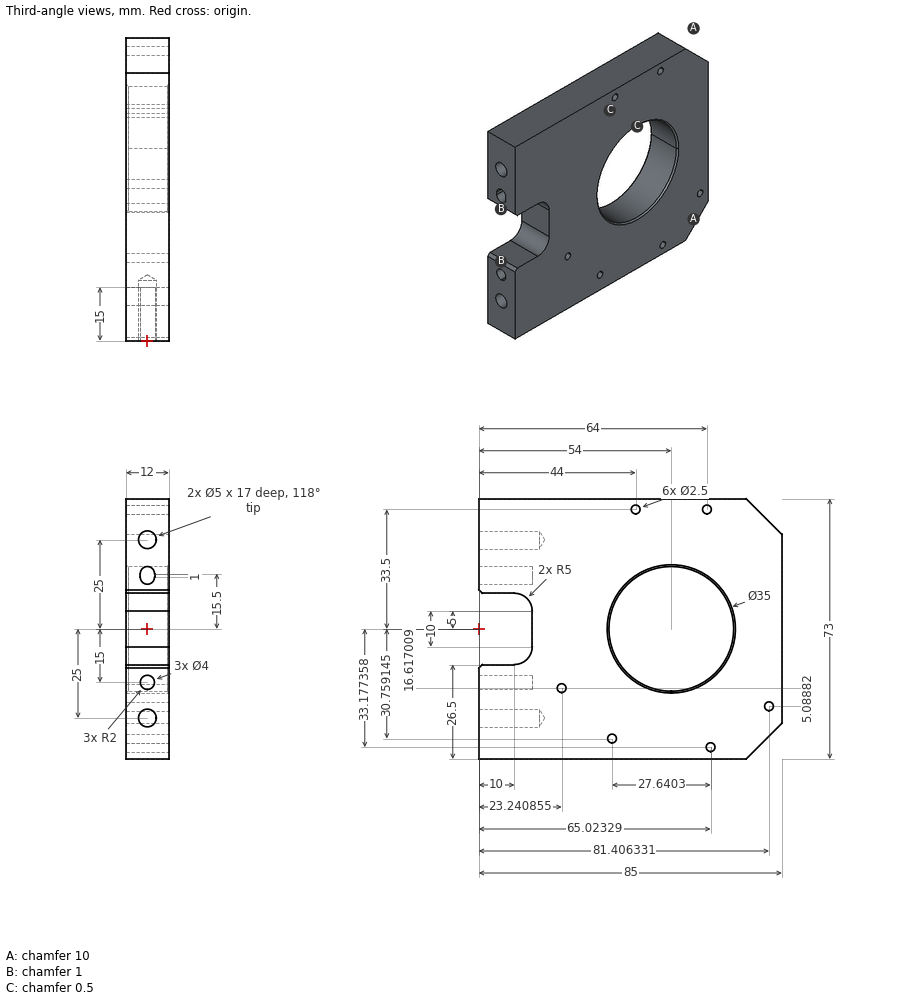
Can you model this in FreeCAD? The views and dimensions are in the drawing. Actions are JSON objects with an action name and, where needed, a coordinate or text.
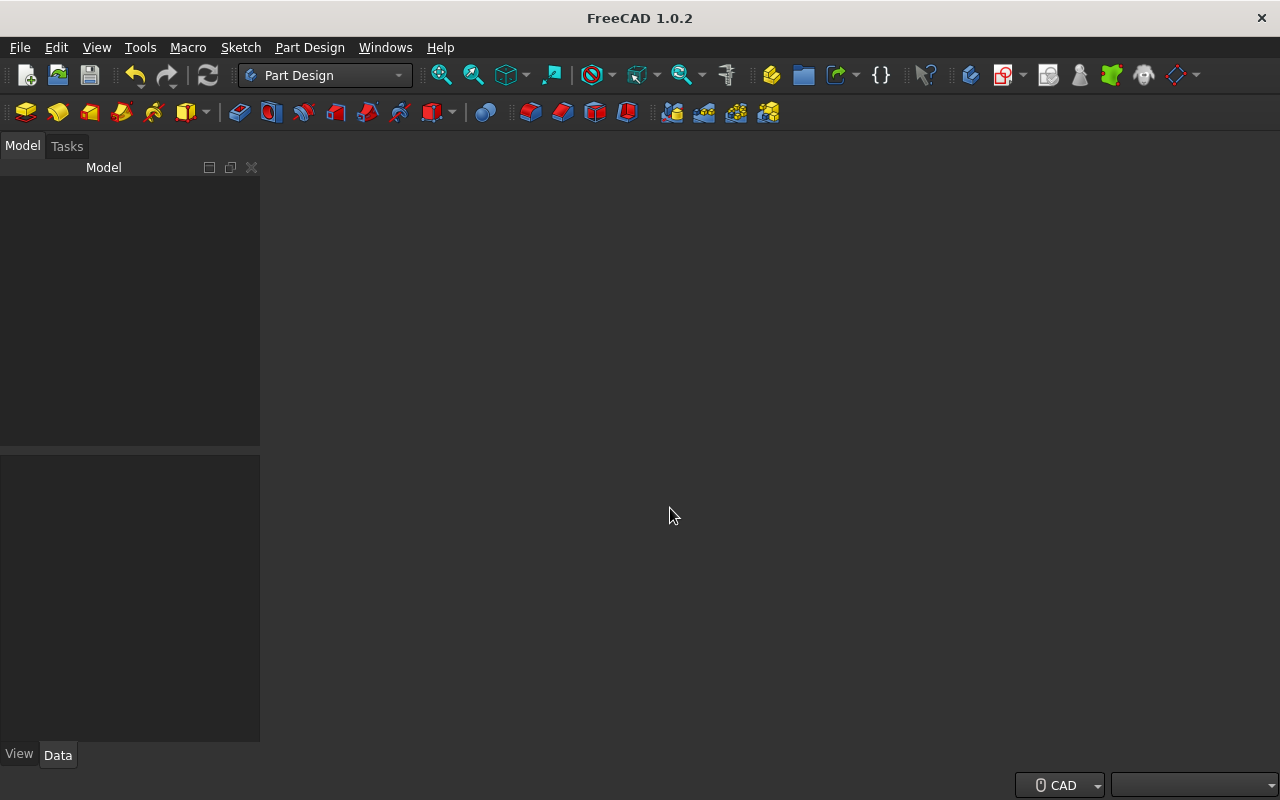
{"action": "left_click", "coordinate": [26, 76]}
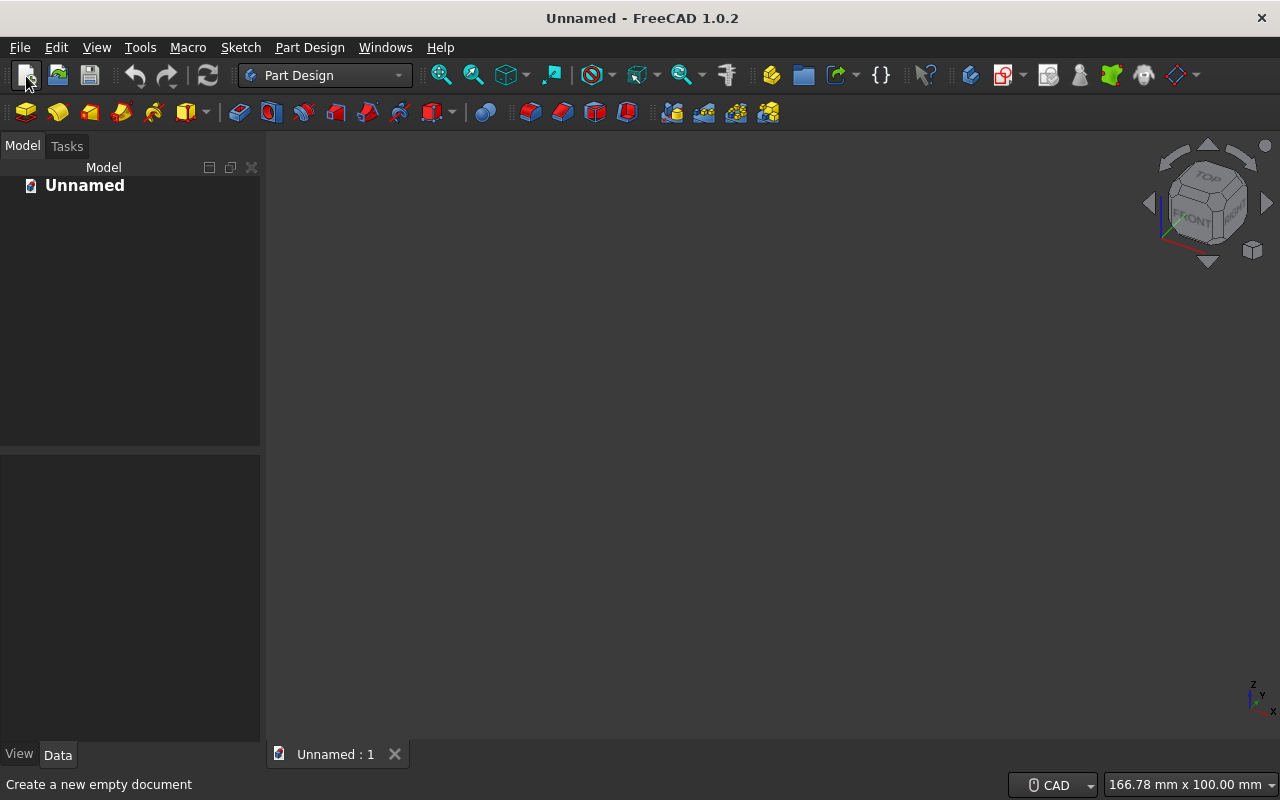
{"action": "left_click", "coordinate": [1004, 76]}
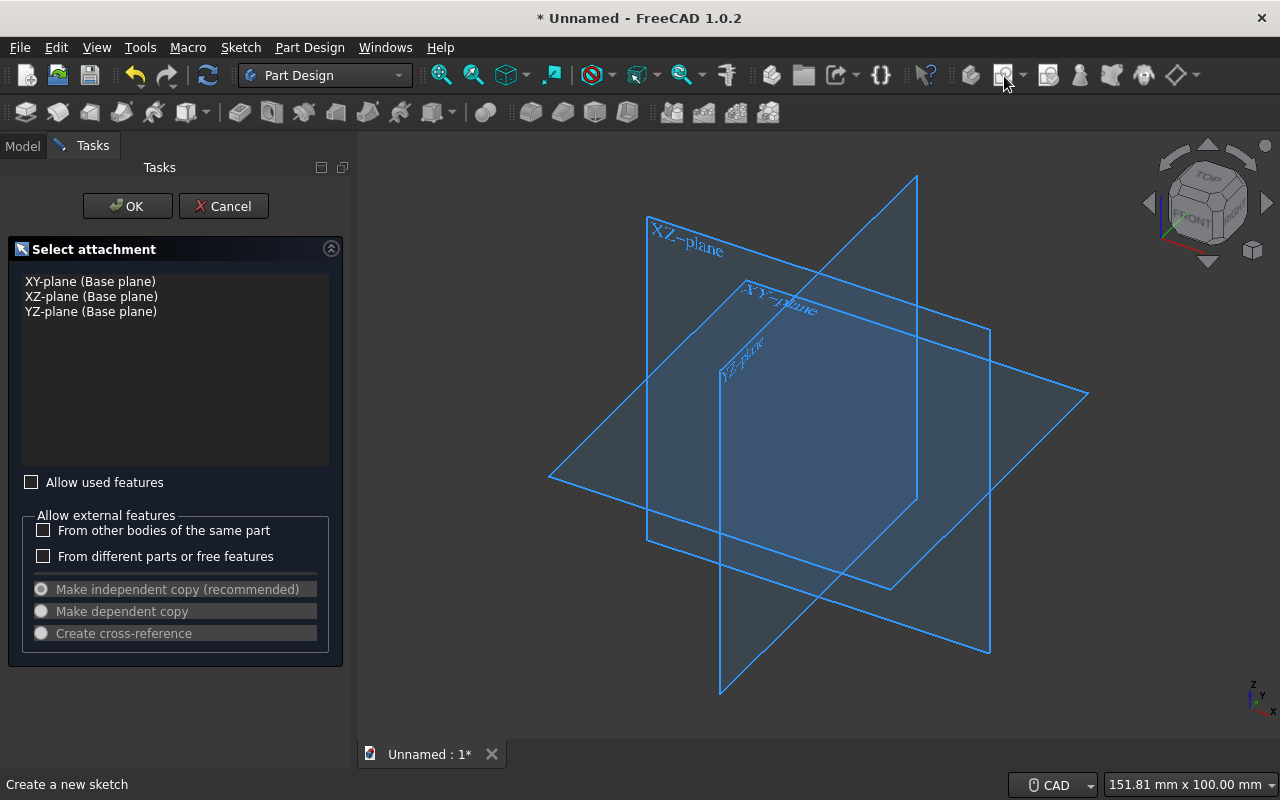
{"action": "left_click", "coordinate": [82, 312]}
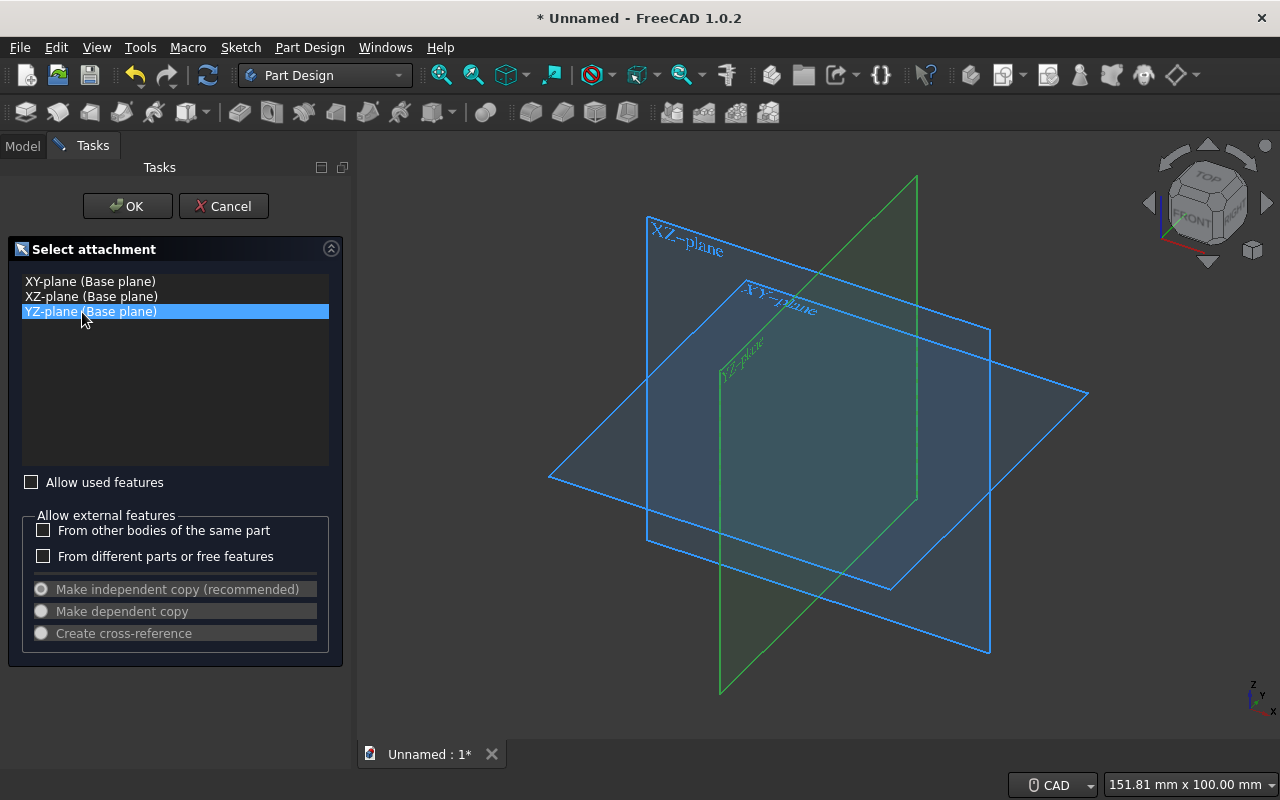
{"action": "left_click", "coordinate": [128, 206]}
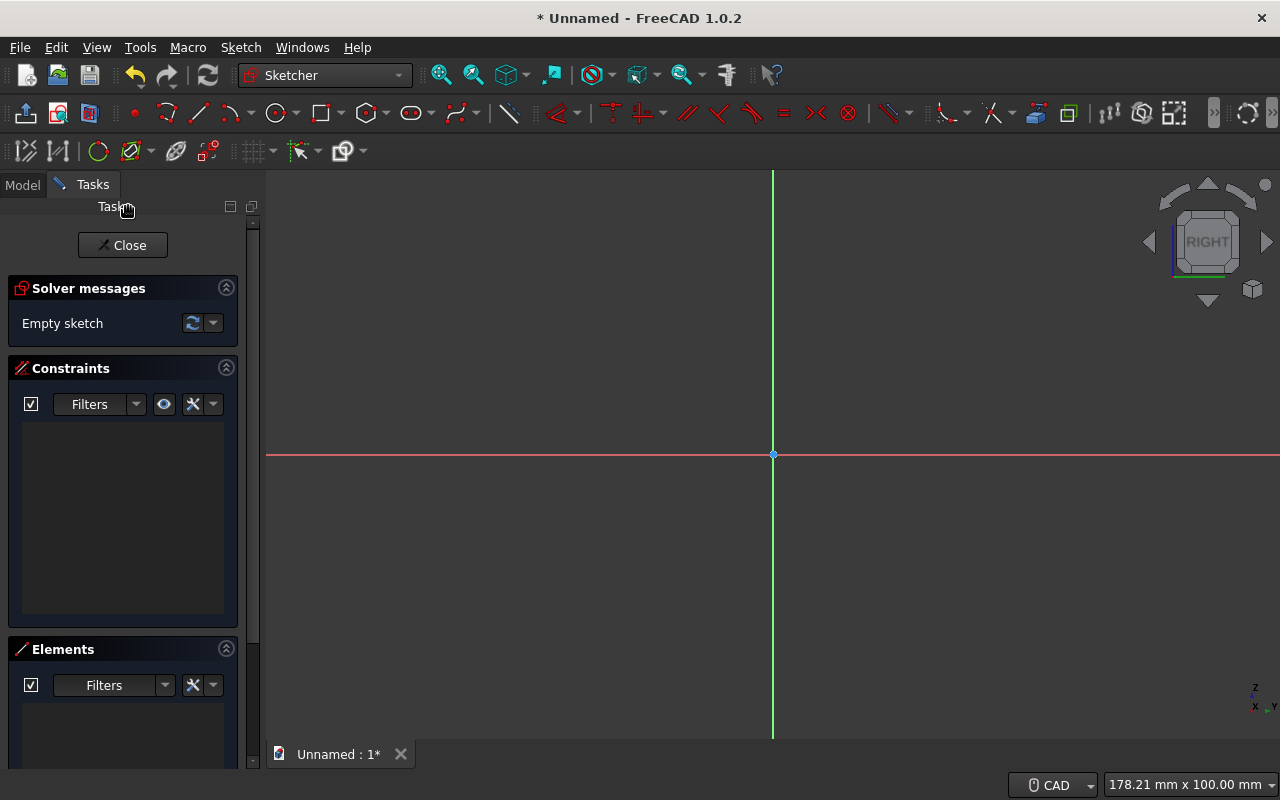
{"action": "scroll", "coordinate": [294, 455], "scroll_direction": "down", "scroll_amount": 1}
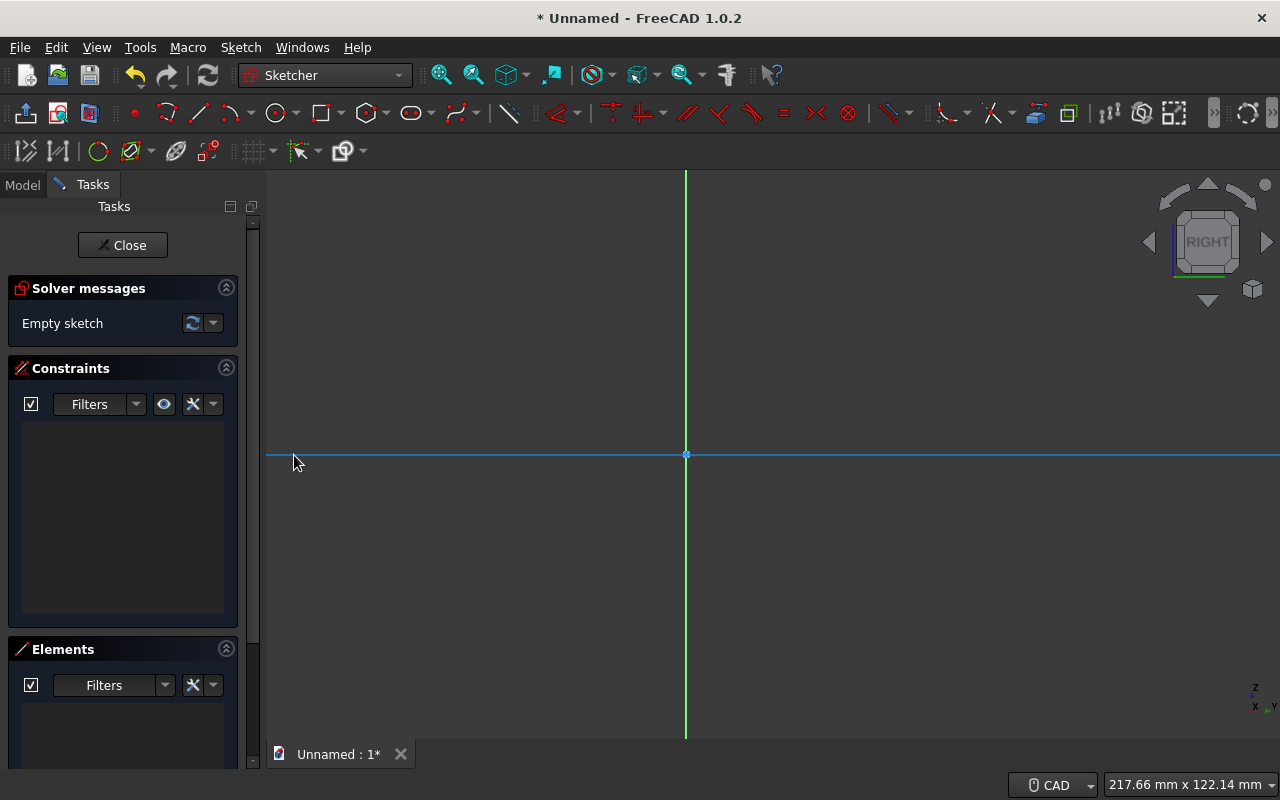
{"action": "left_click", "coordinate": [200, 114]}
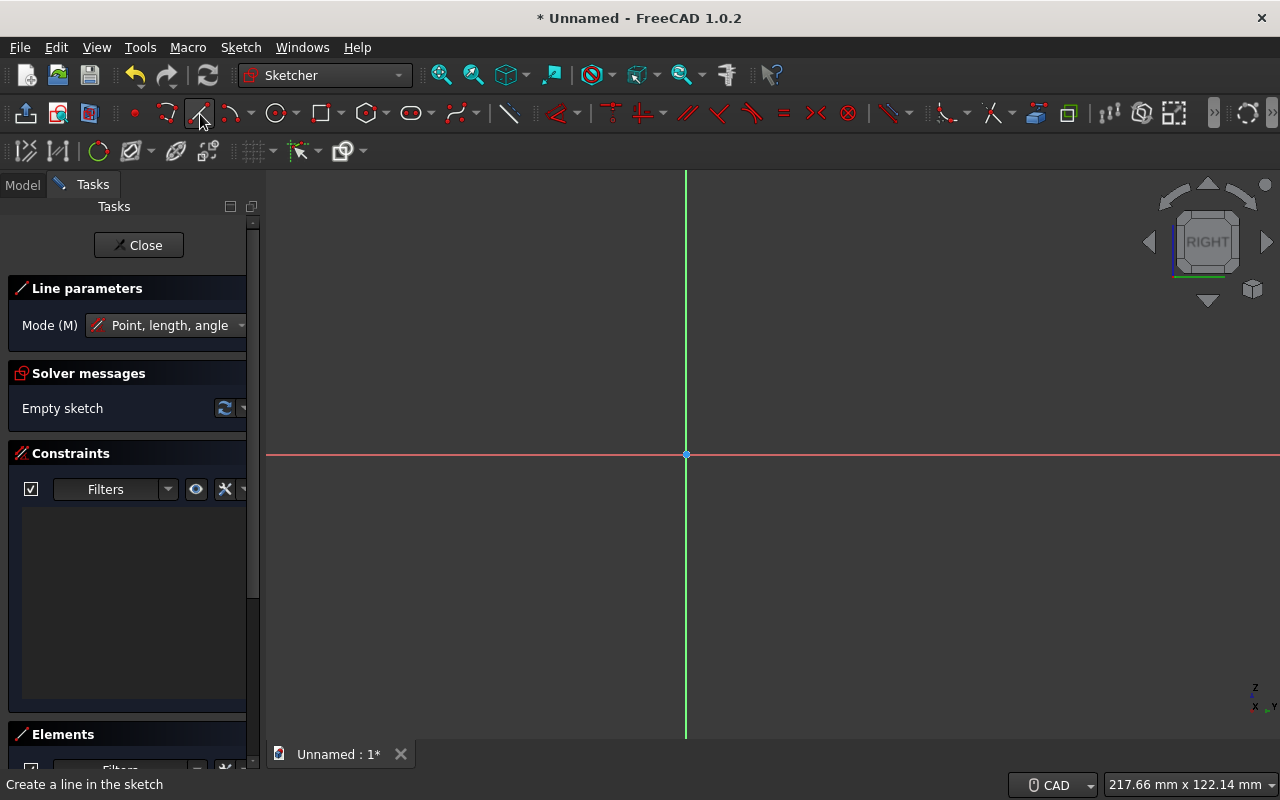
{"action": "left_click", "coordinate": [756, 431]}
{"action": "left_click", "coordinate": [756, 478]}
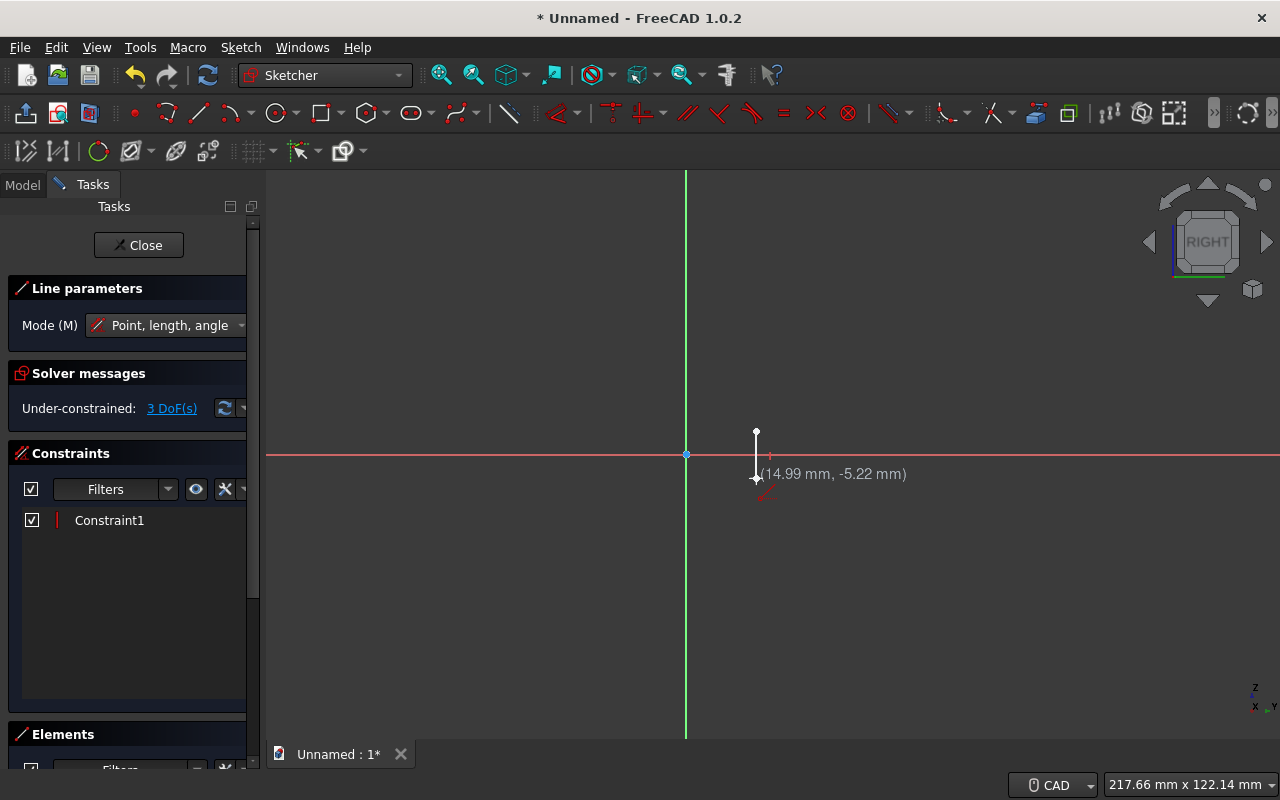
{"action": "left_click", "coordinate": [168, 114]}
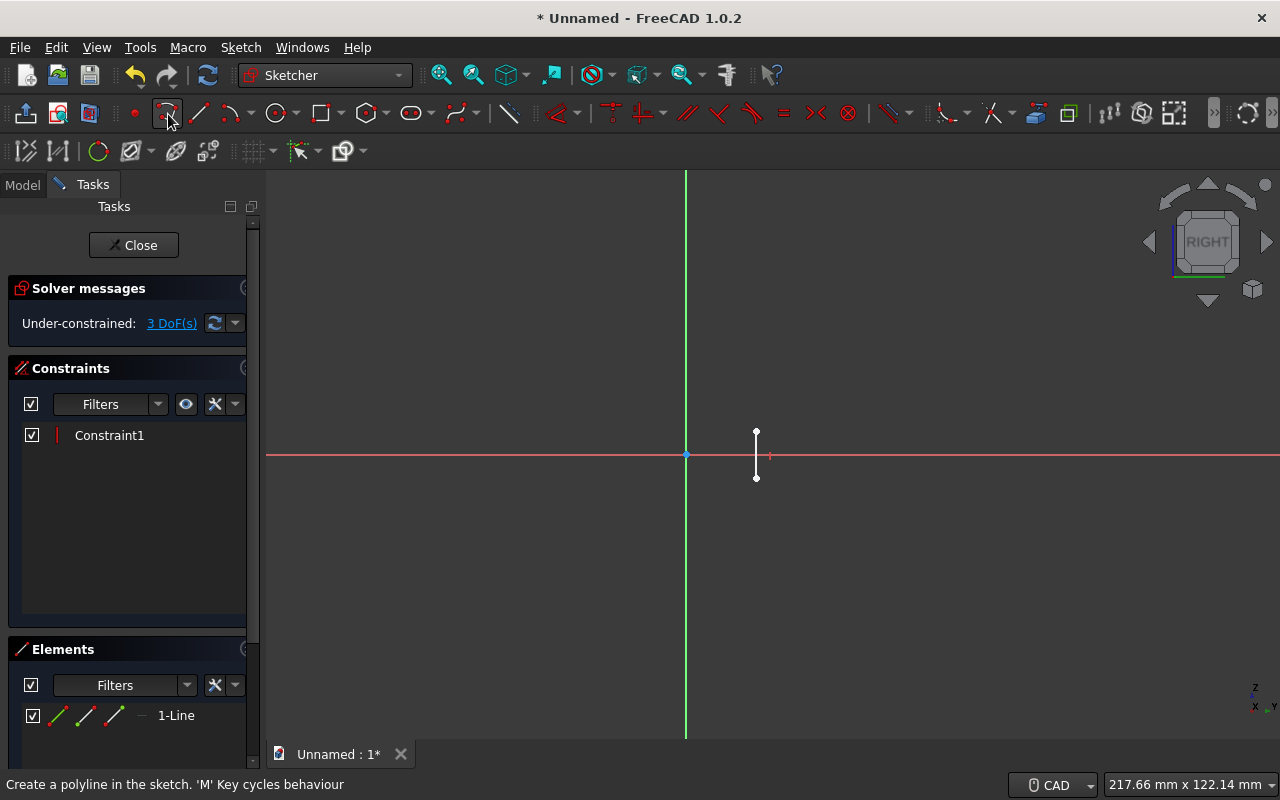
{"action": "left_click", "coordinate": [733, 501]}
{"action": "left_click", "coordinate": [686, 501]}
{"action": "left_click", "coordinate": [695, 625]}
{"action": "left_click", "coordinate": [1082, 625]}
{"action": "left_click", "coordinate": [1082, 285]}
{"action": "left_click", "coordinate": [686, 285]}
{"action": "left_click", "coordinate": [695, 408]}
{"action": "left_click", "coordinate": [733, 408]}
{"action": "right_click", "coordinate": [733, 408]}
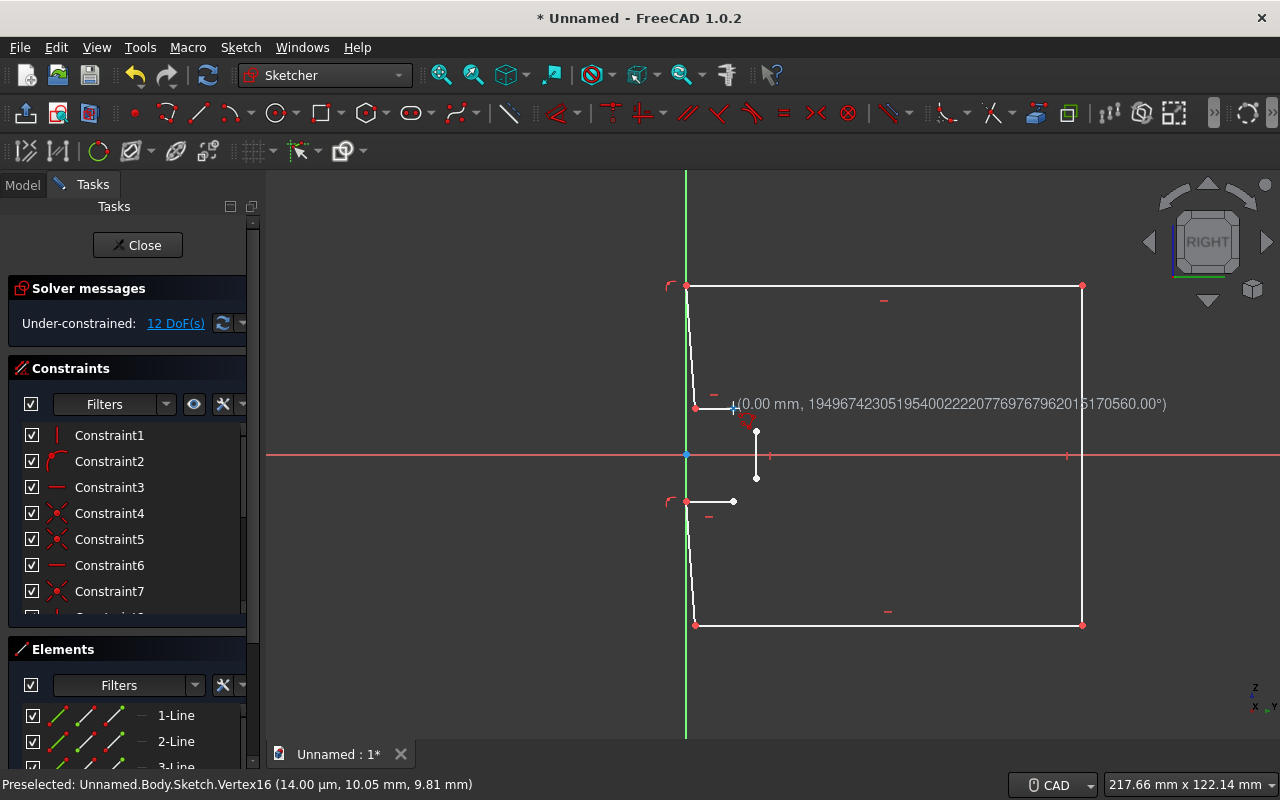
{"action": "left_click", "coordinate": [254, 114]}